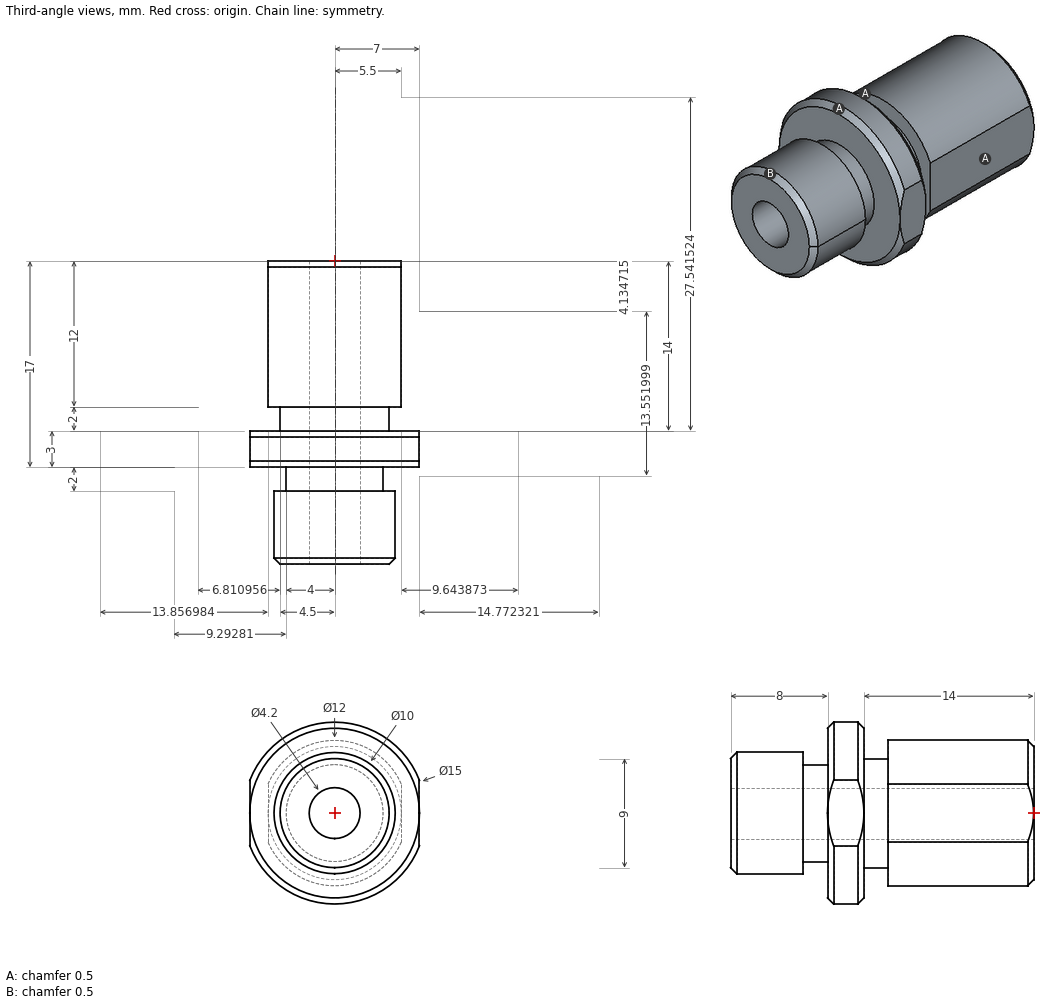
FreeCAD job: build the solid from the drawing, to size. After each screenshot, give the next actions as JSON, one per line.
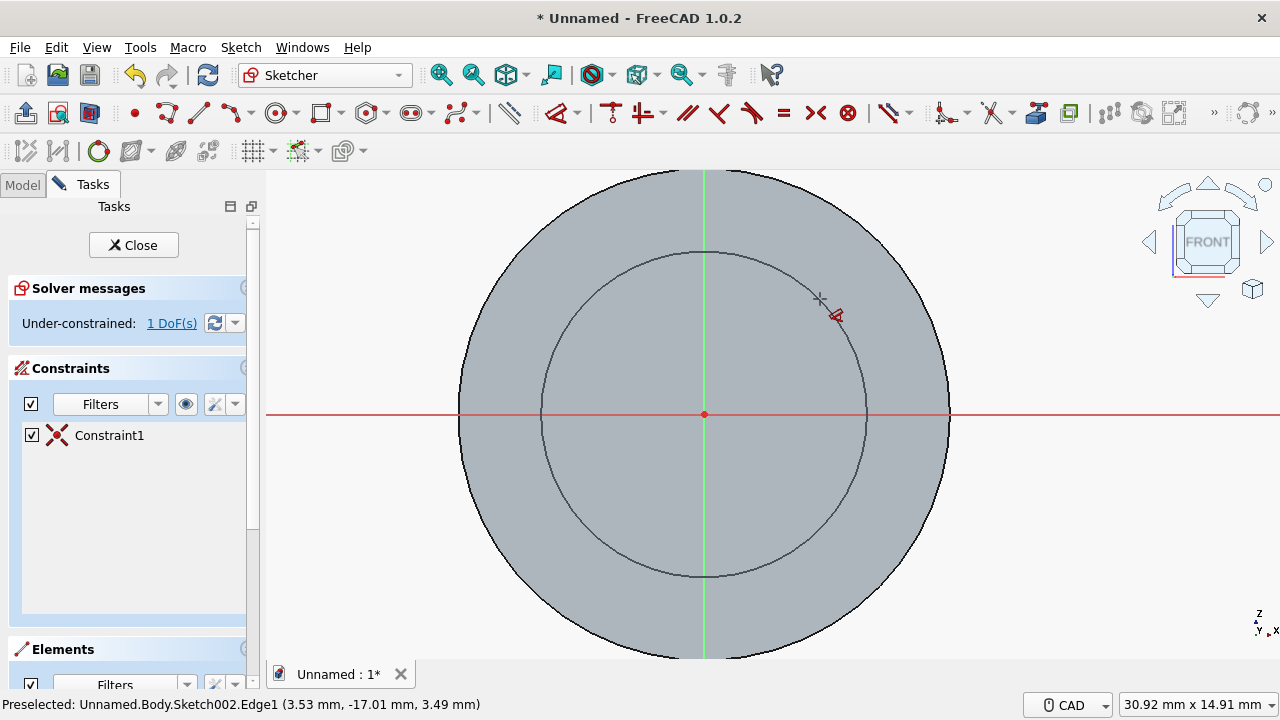
{"action": "left_click", "coordinate": [819, 299]}
{"action": "left_click", "coordinate": [842, 276]}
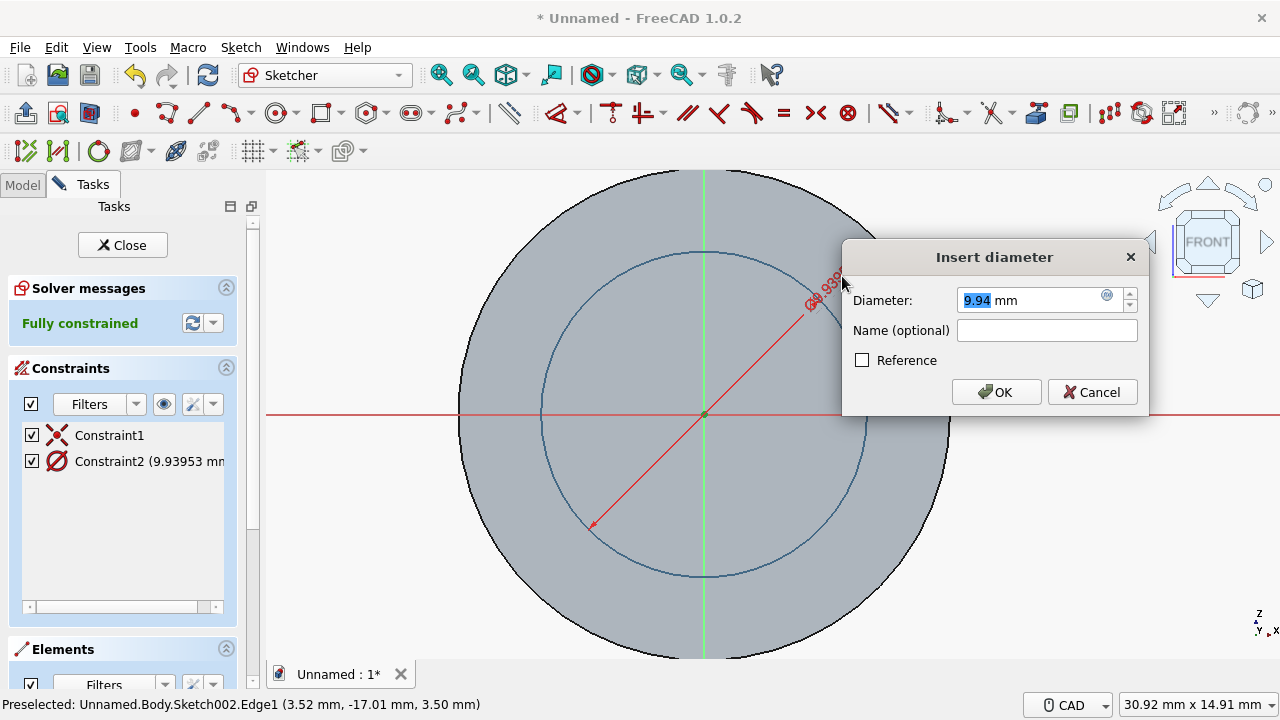
{"action": "type", "text": "10"}
{"action": "key", "text": "Return"}
{"action": "key", "text": "Escape"}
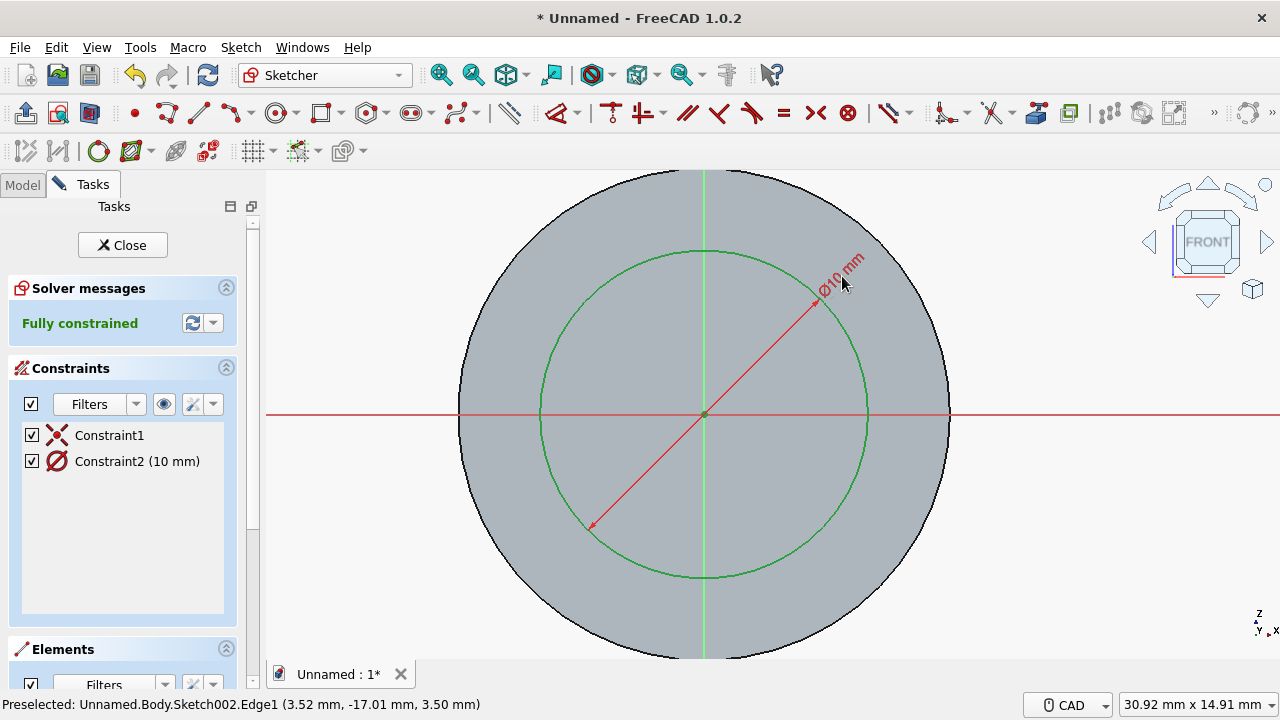
{"action": "left_click", "coordinate": [123, 245]}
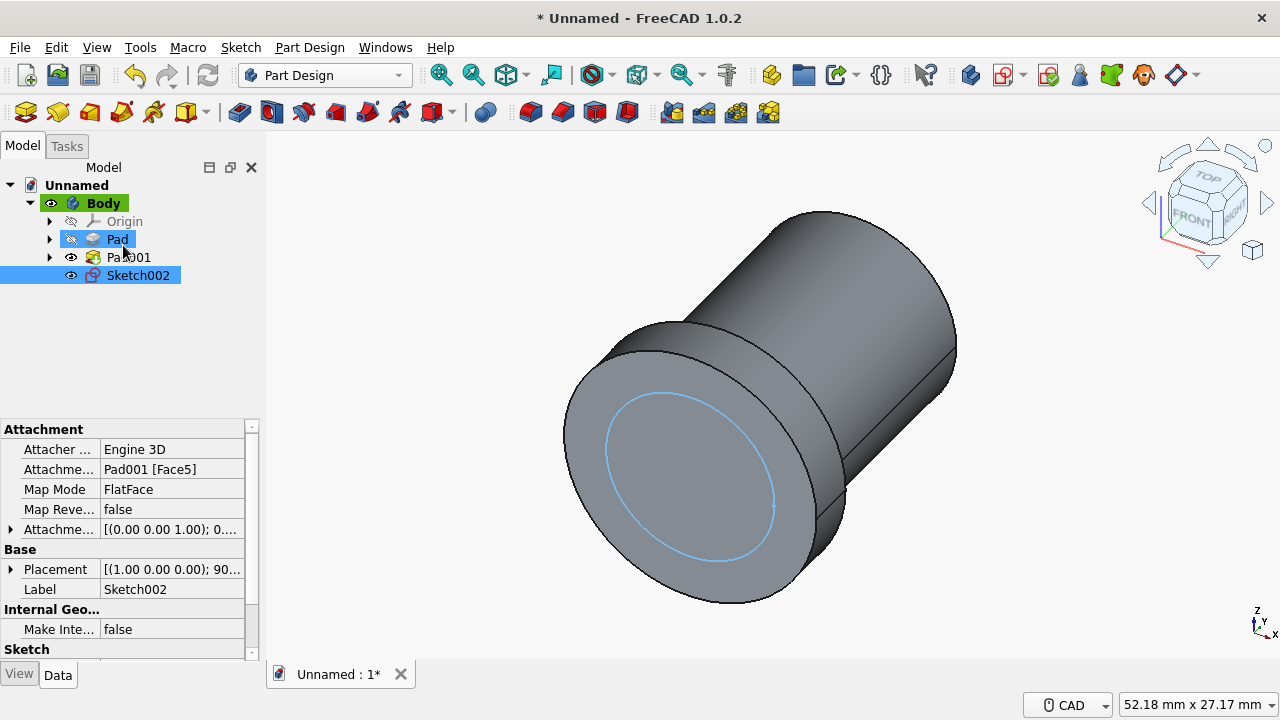
{"action": "left_click", "coordinate": [26, 112]}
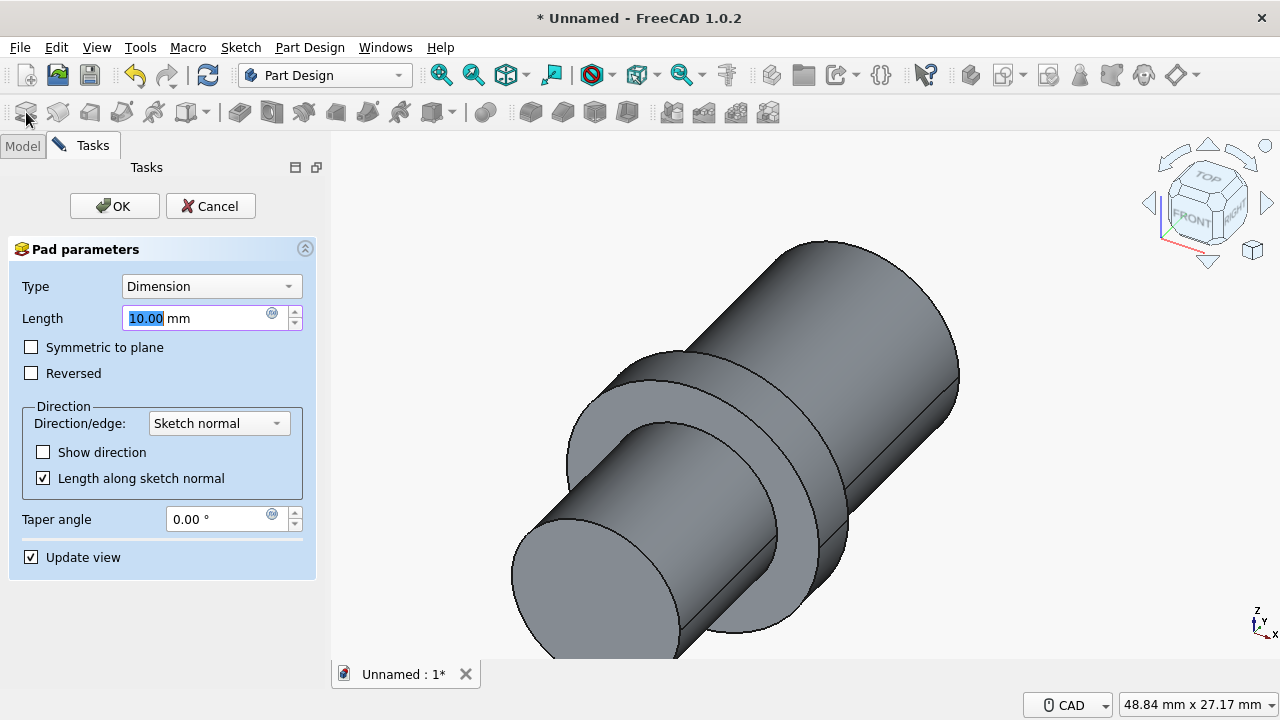
{"action": "type", "text": "8"}
{"action": "key", "text": "Tab"}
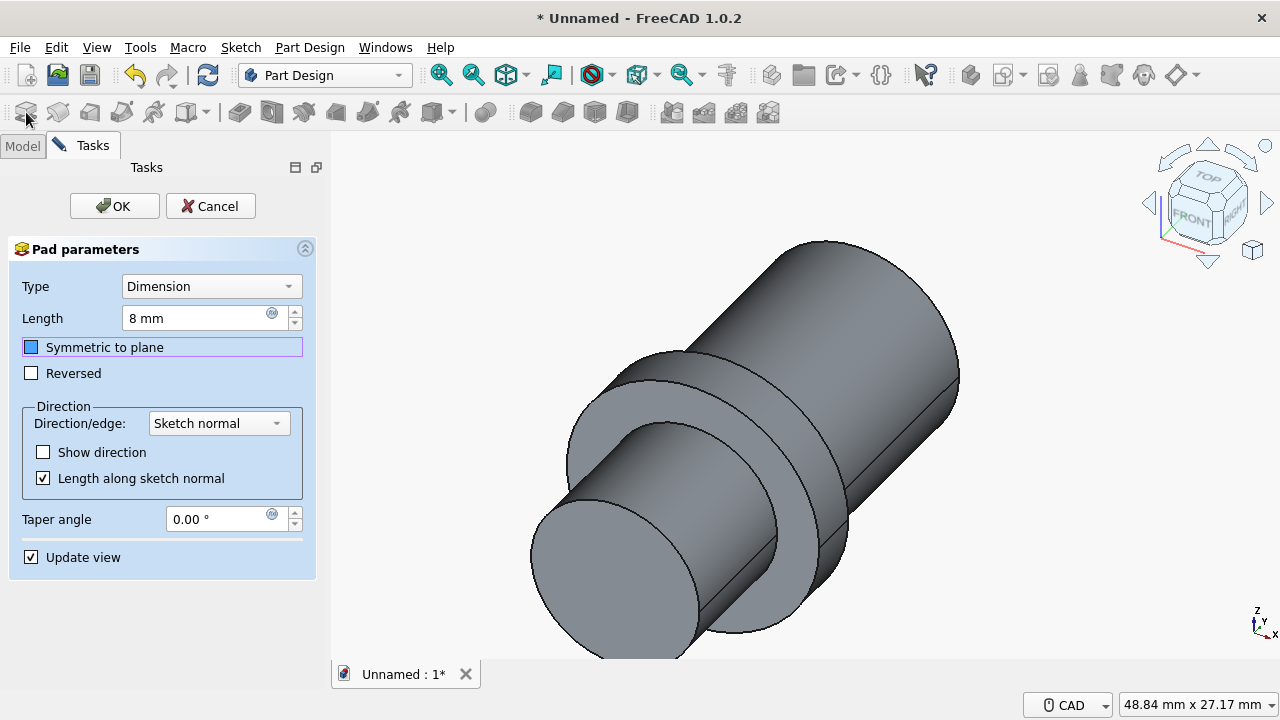
{"action": "left_click", "coordinate": [115, 206]}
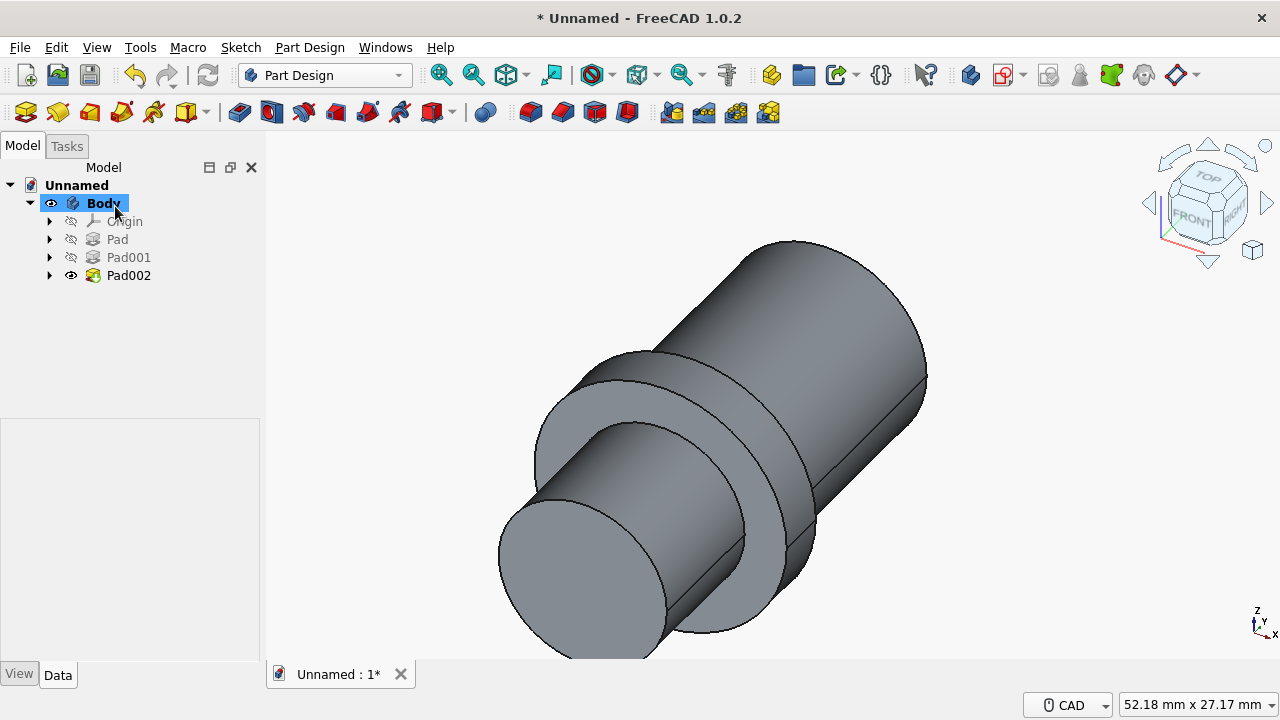
{"action": "key", "text": "v f"}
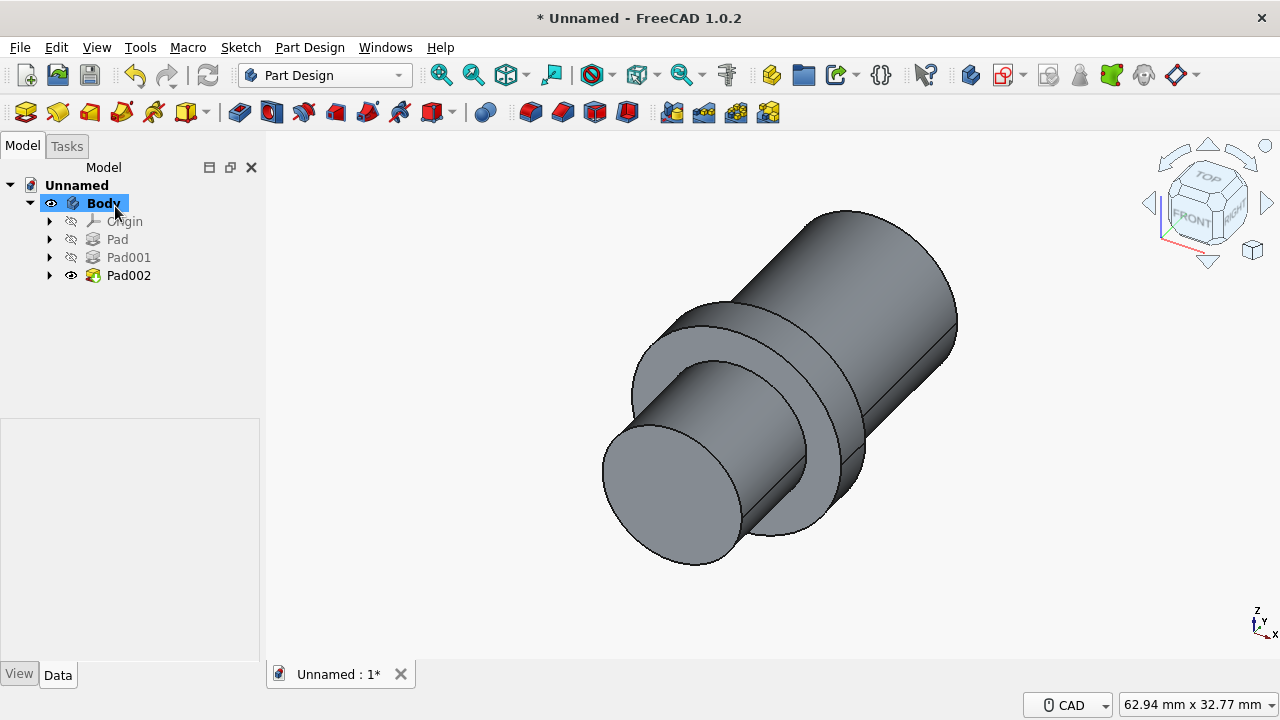
{"action": "left_click", "coordinate": [1004, 76]}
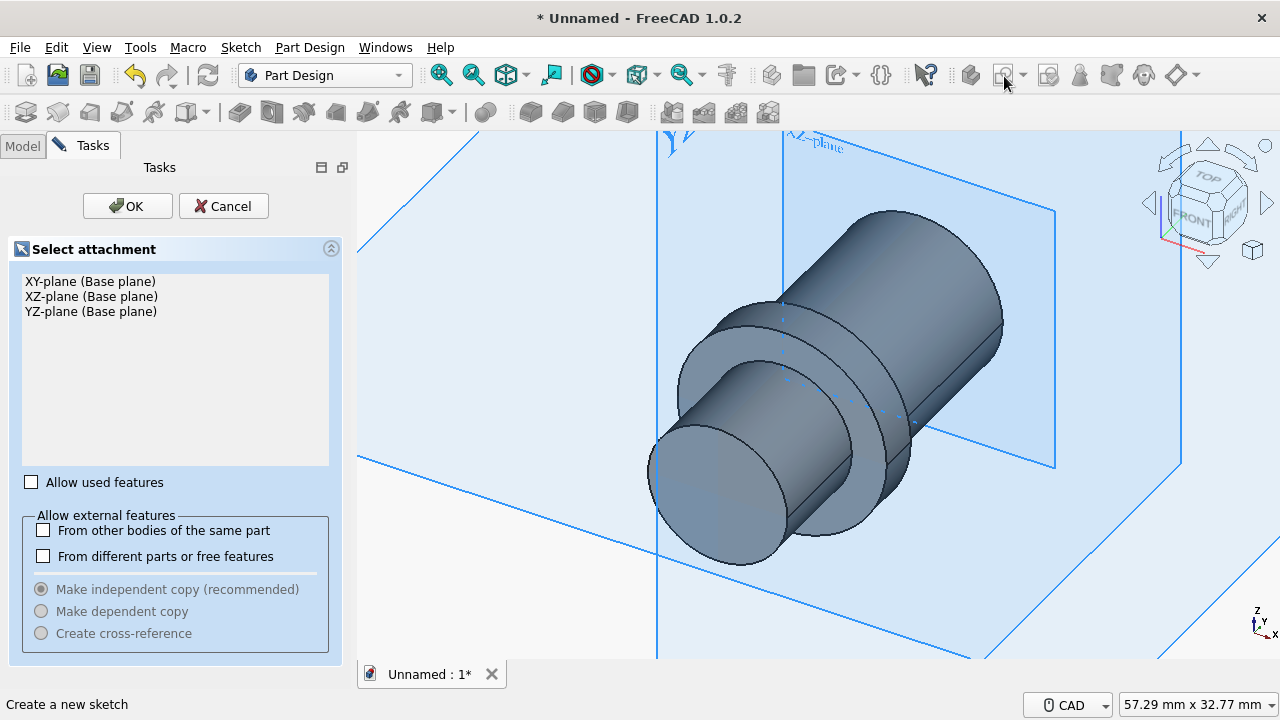
{"action": "left_click", "coordinate": [82, 296]}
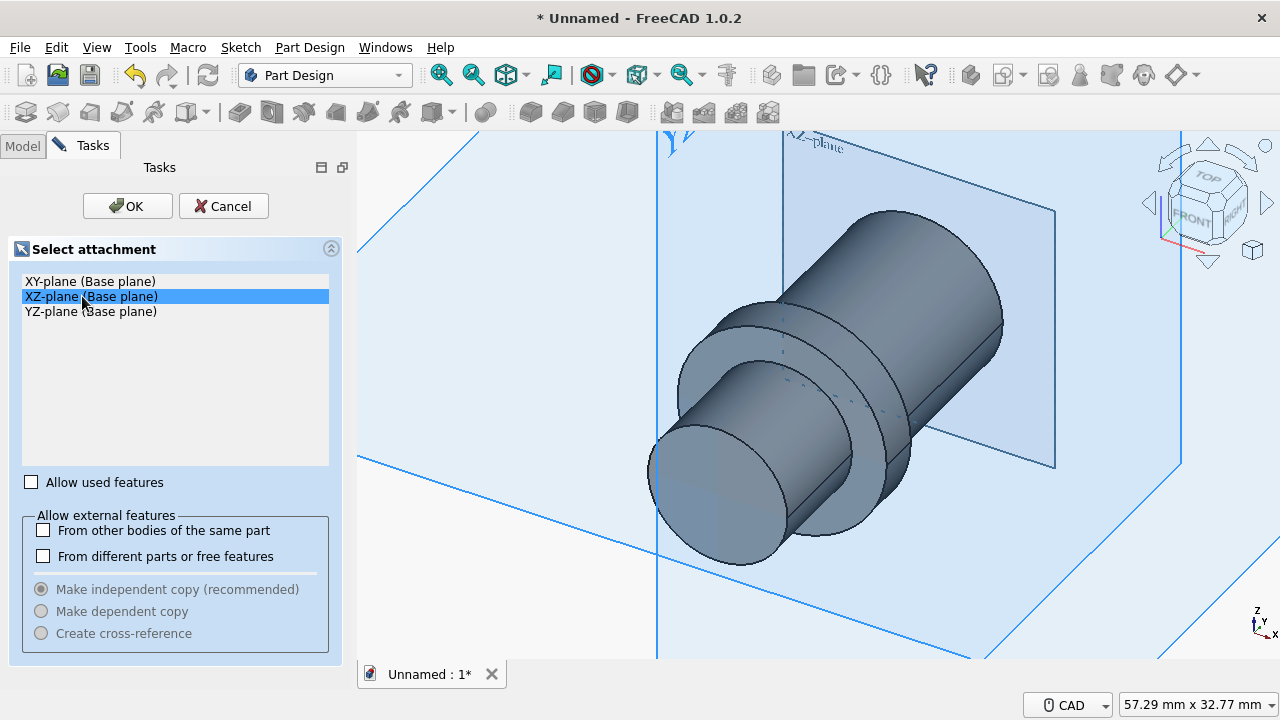
{"action": "left_click", "coordinate": [128, 206]}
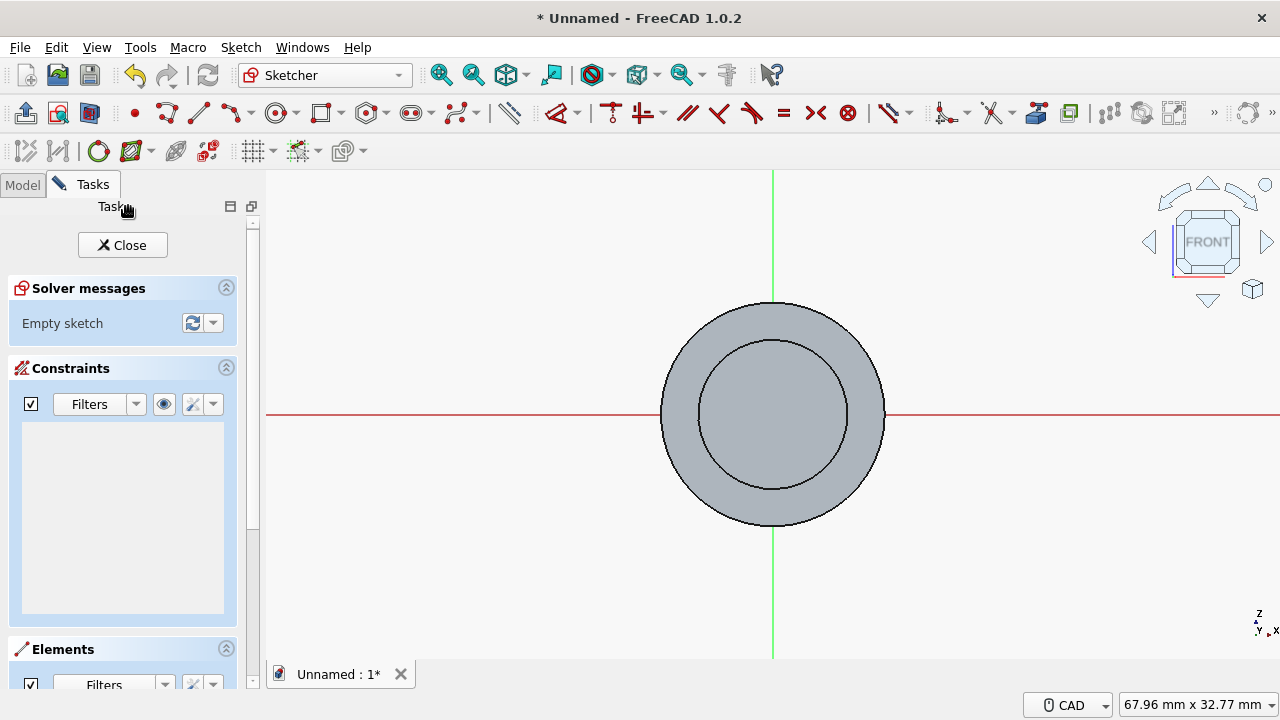
{"action": "left_click", "coordinate": [90, 114]}